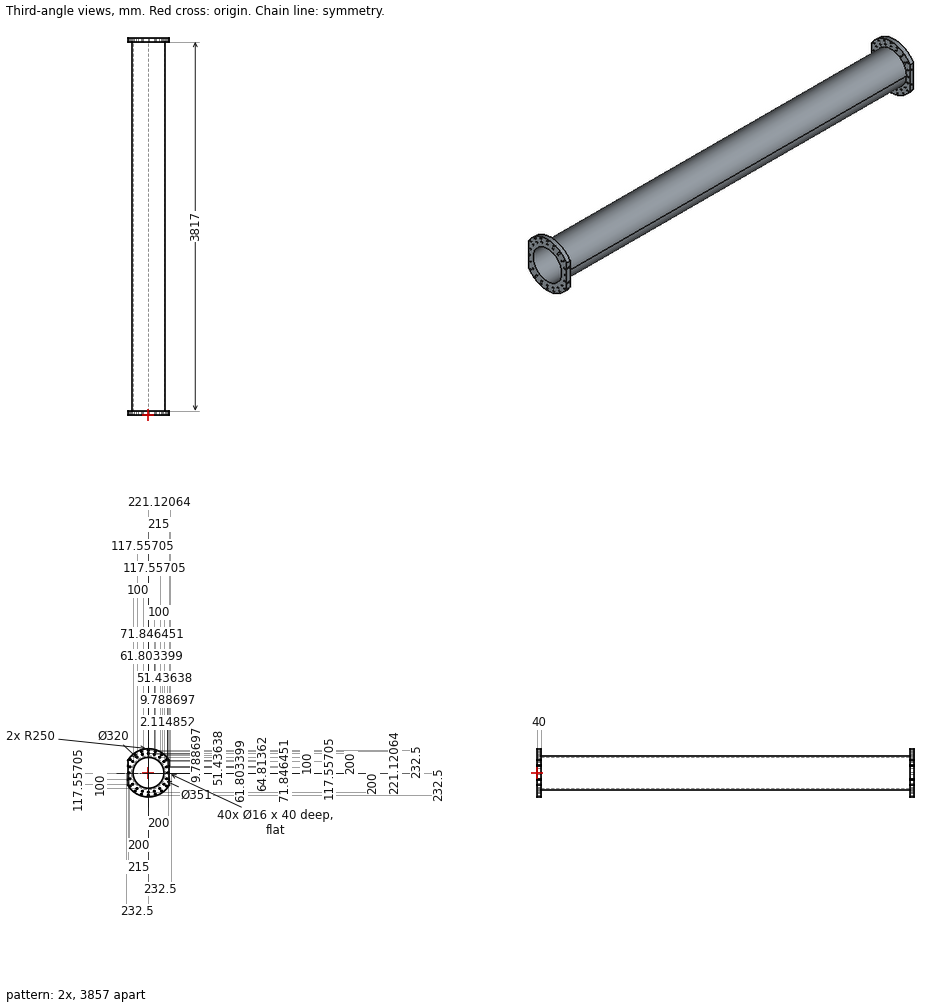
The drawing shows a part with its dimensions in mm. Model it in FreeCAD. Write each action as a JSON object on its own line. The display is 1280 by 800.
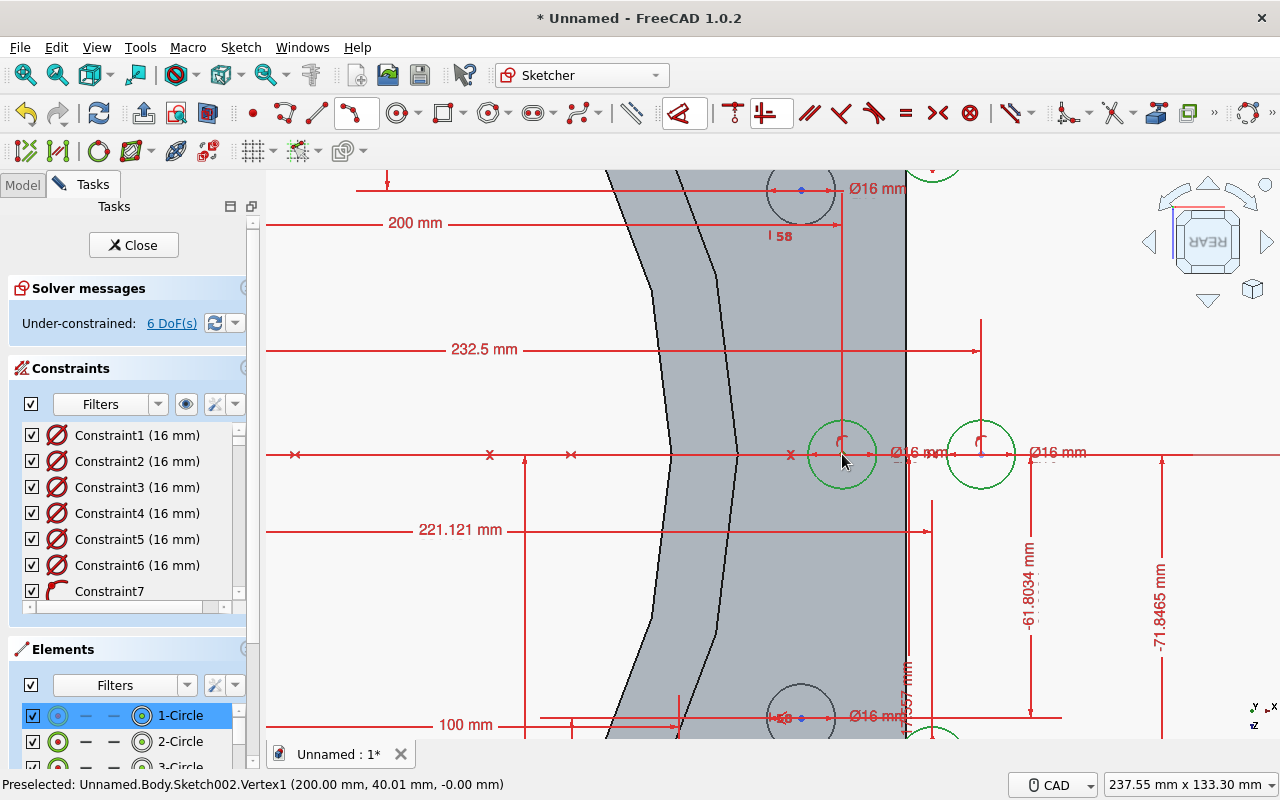
{"action": "scroll", "coordinate": [846, 455], "scroll_direction": "down", "scroll_amount": 9}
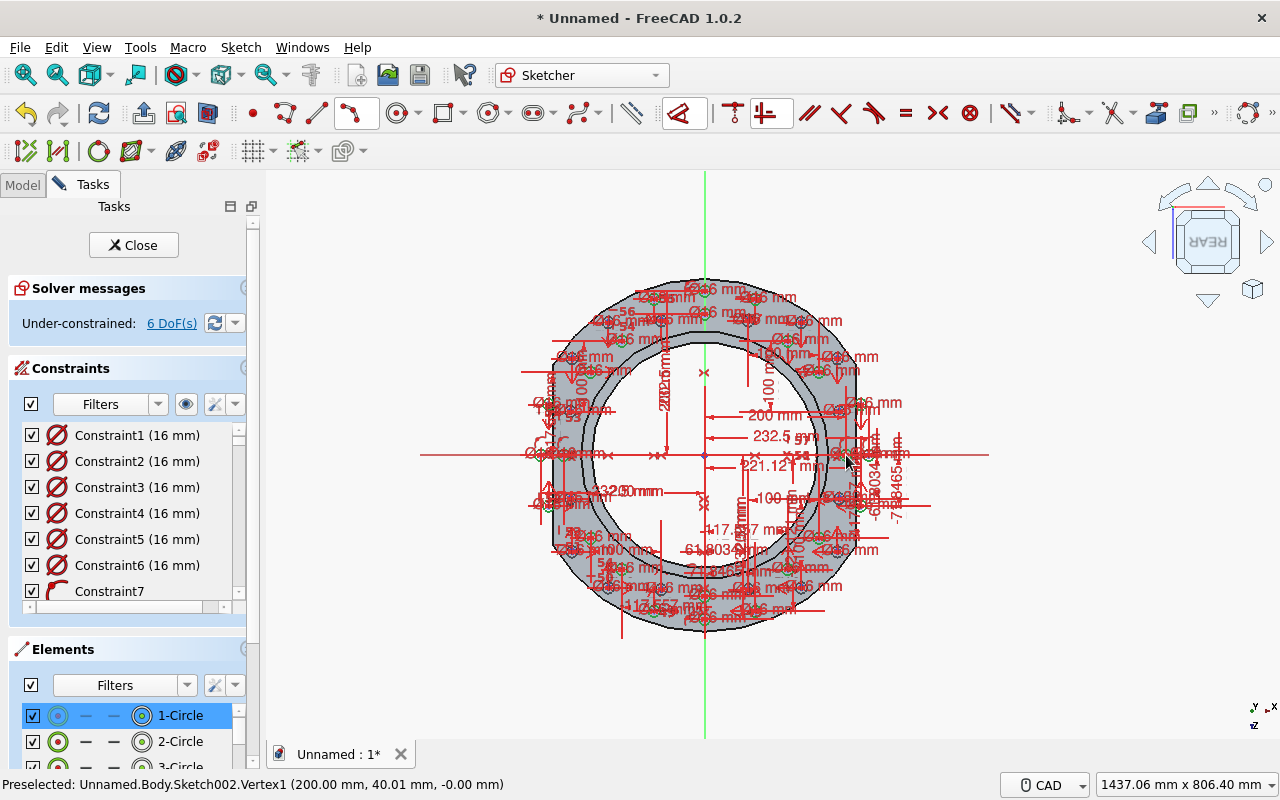
{"action": "scroll", "coordinate": [839, 499], "scroll_direction": "up", "scroll_amount": 9}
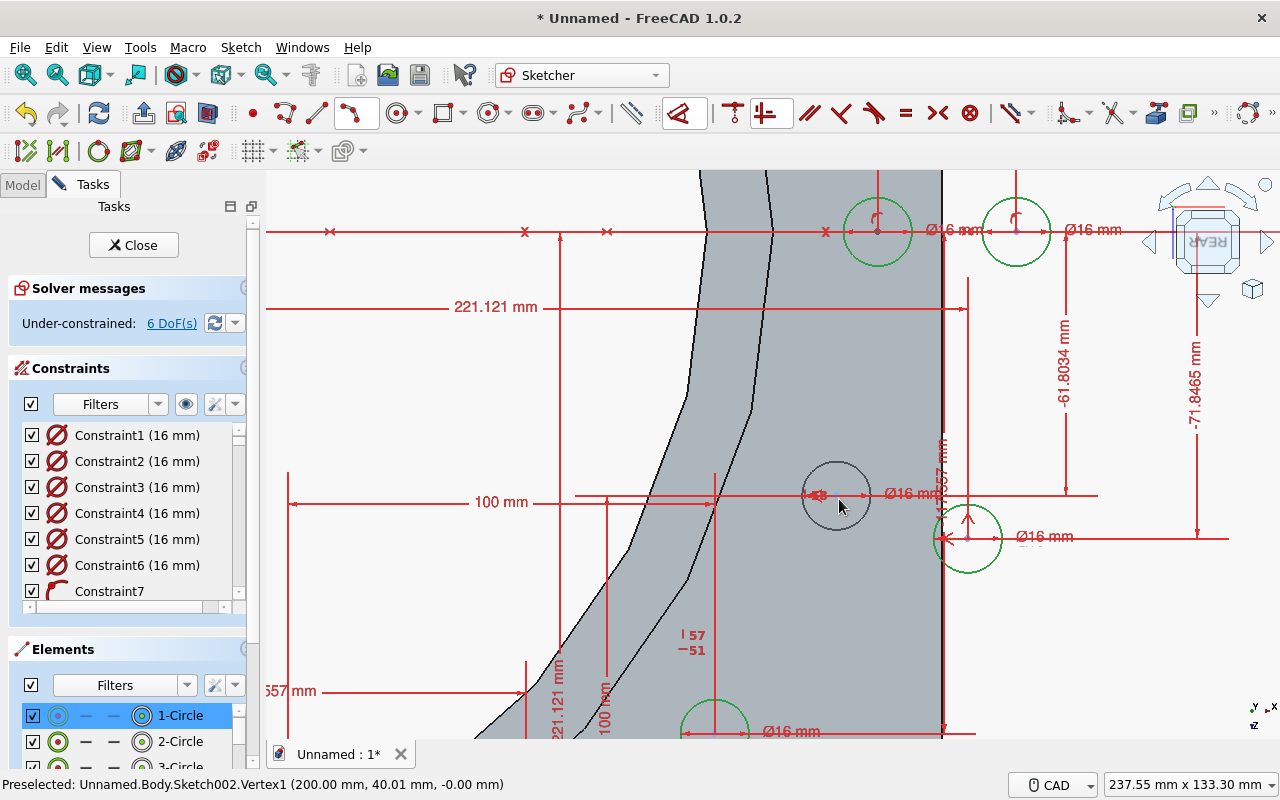
{"action": "left_click", "coordinate": [836, 496]}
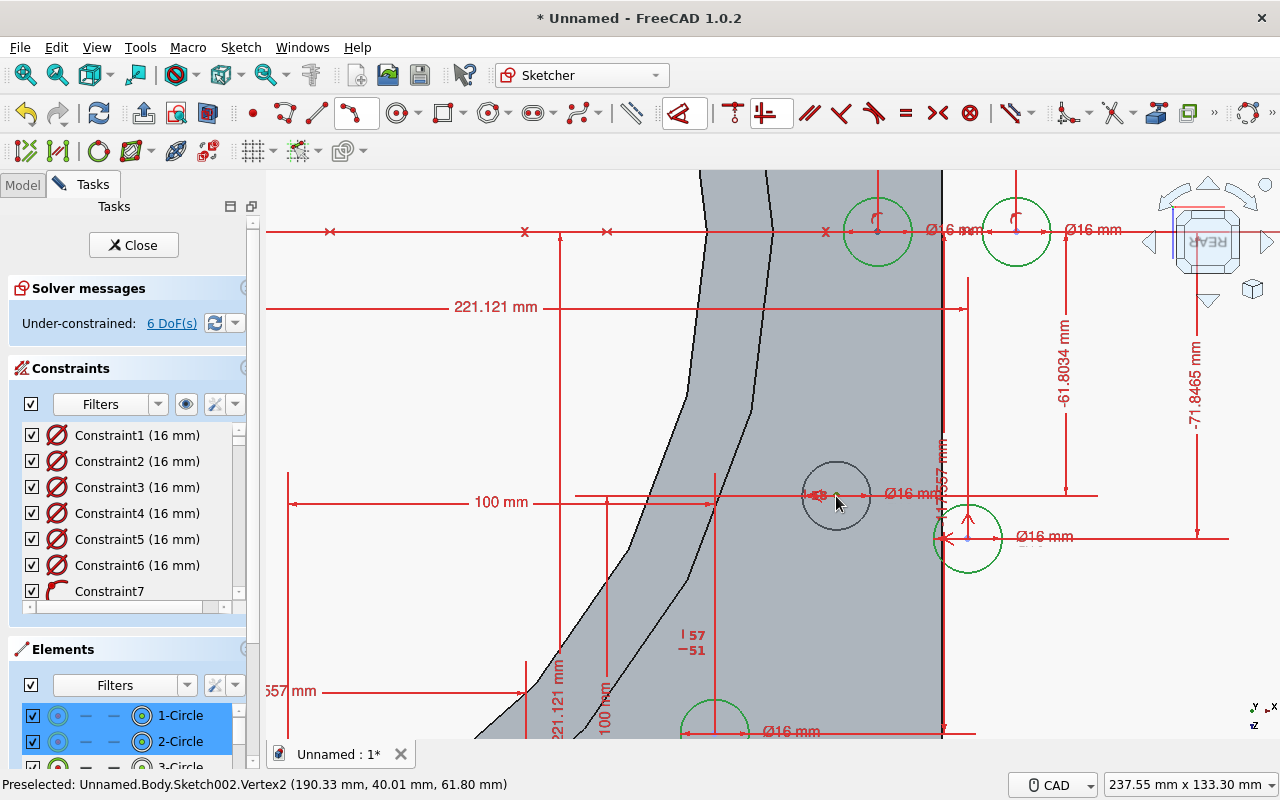
{"action": "left_click", "coordinate": [702, 114]}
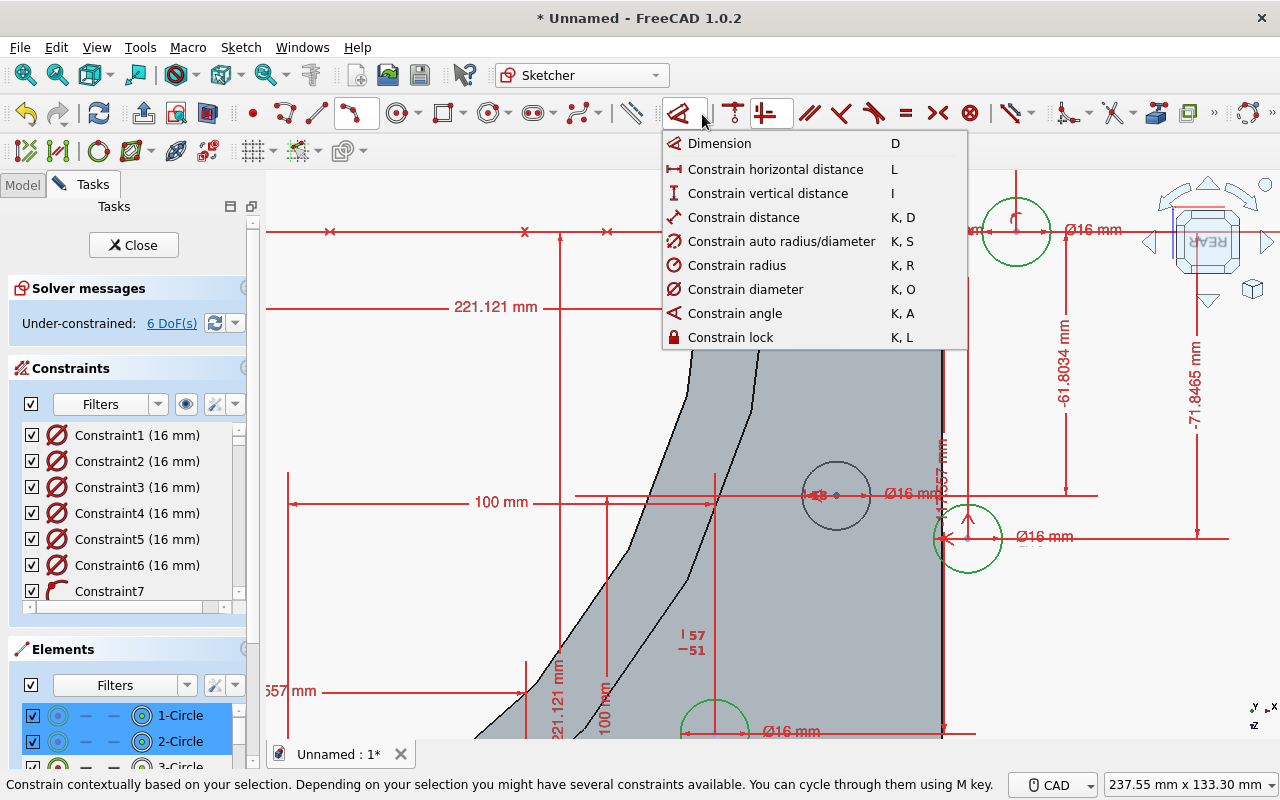
{"action": "left_click", "coordinate": [815, 169]}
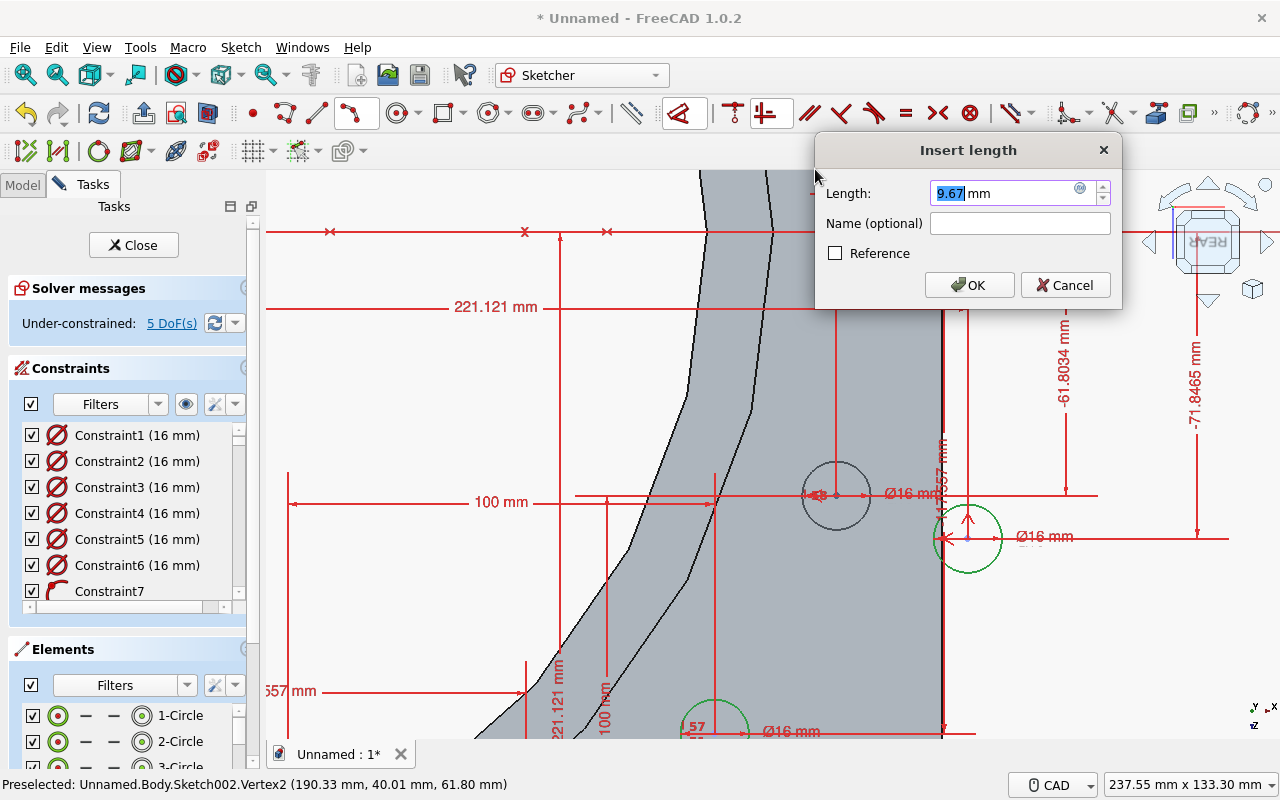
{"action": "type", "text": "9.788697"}
{"action": "key", "text": "Return"}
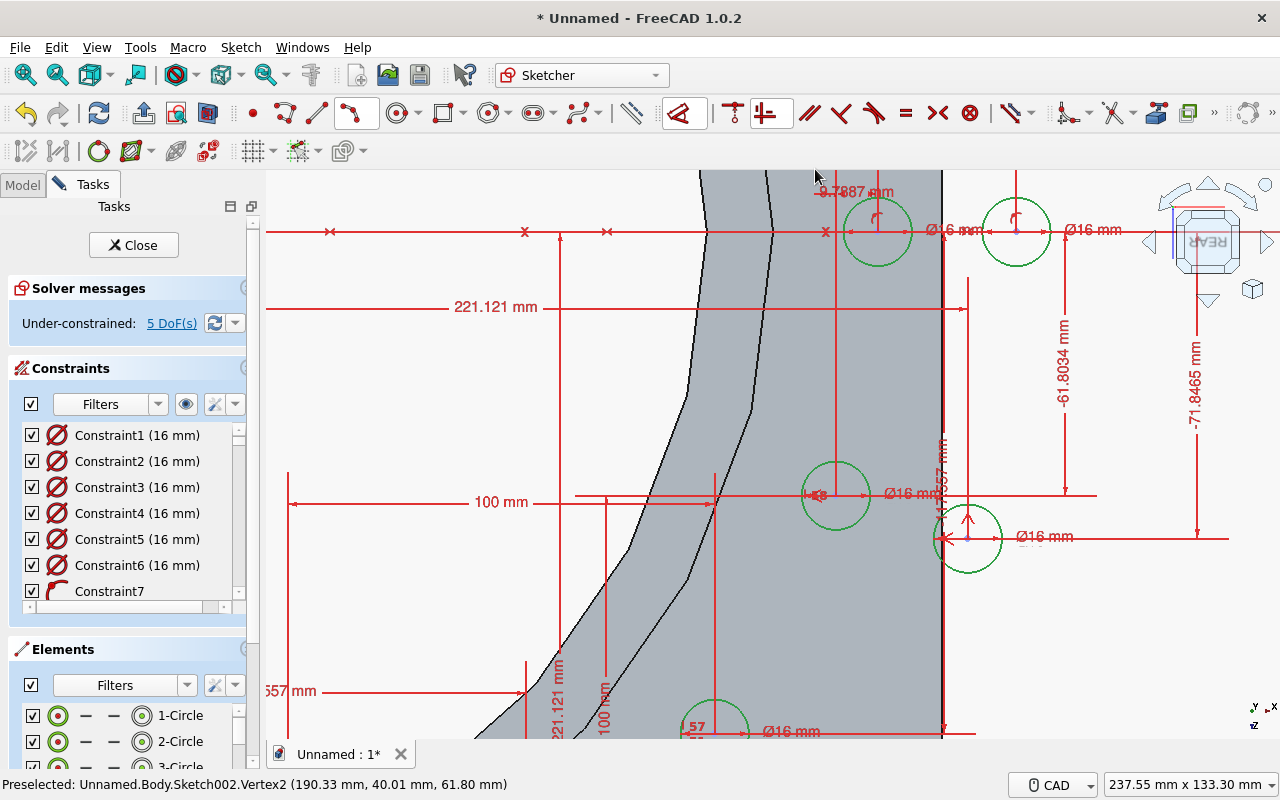
{"action": "scroll", "coordinate": [839, 499], "scroll_direction": "down", "scroll_amount": 9}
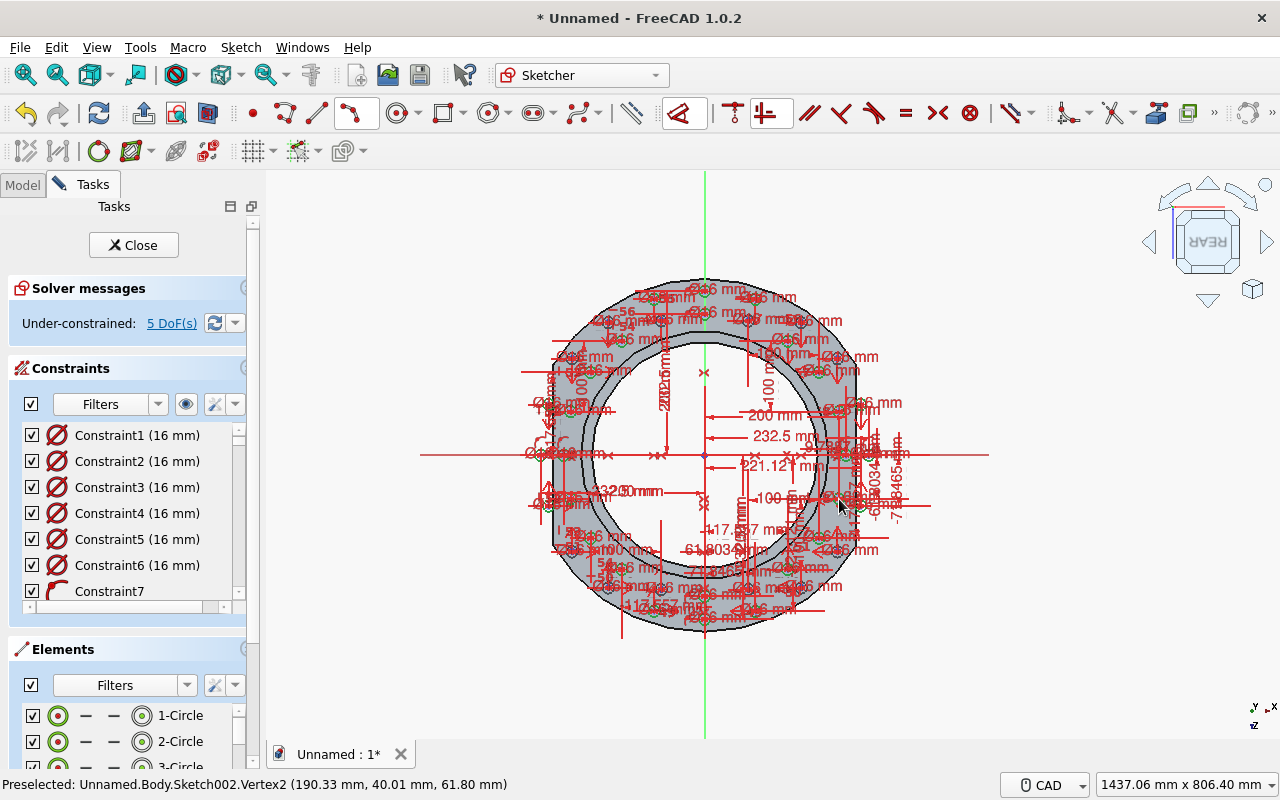
{"action": "scroll", "coordinate": [748, 590], "scroll_direction": "up", "scroll_amount": 9}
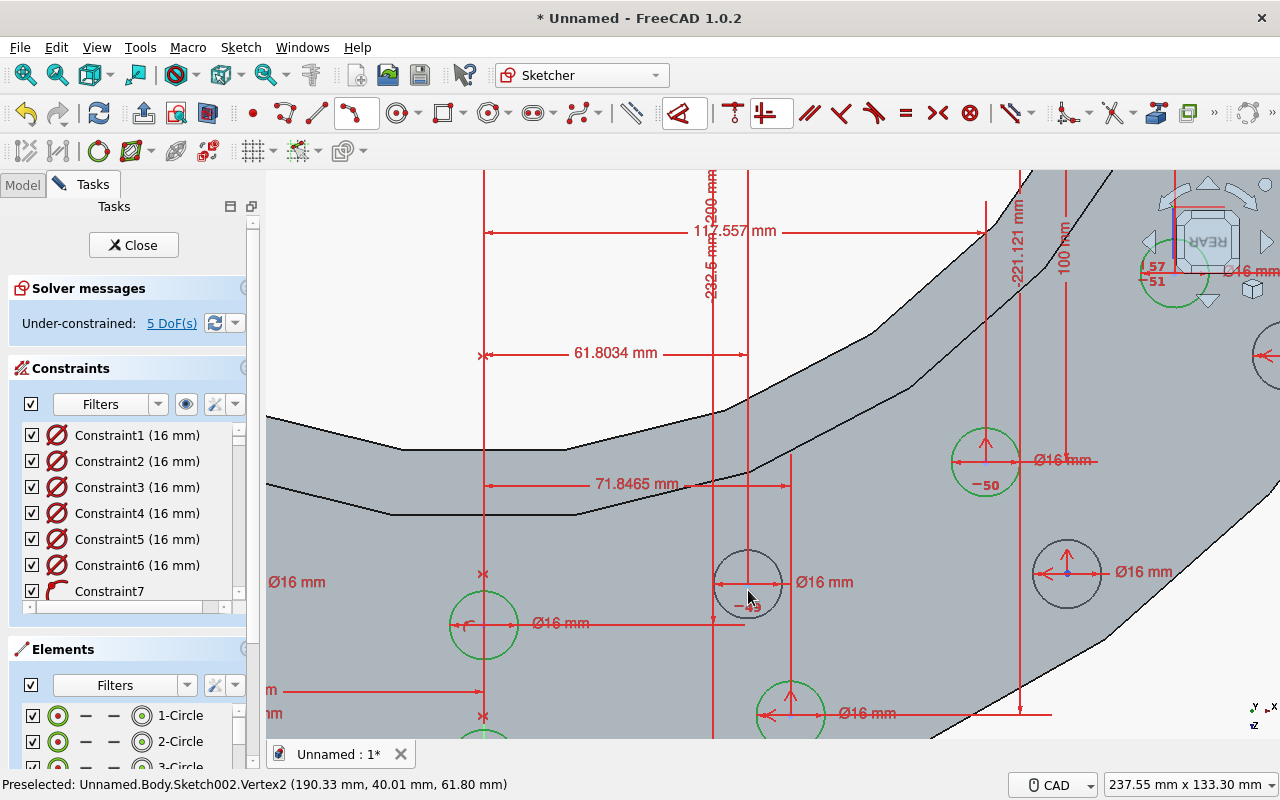
{"action": "left_click", "coordinate": [748, 584]}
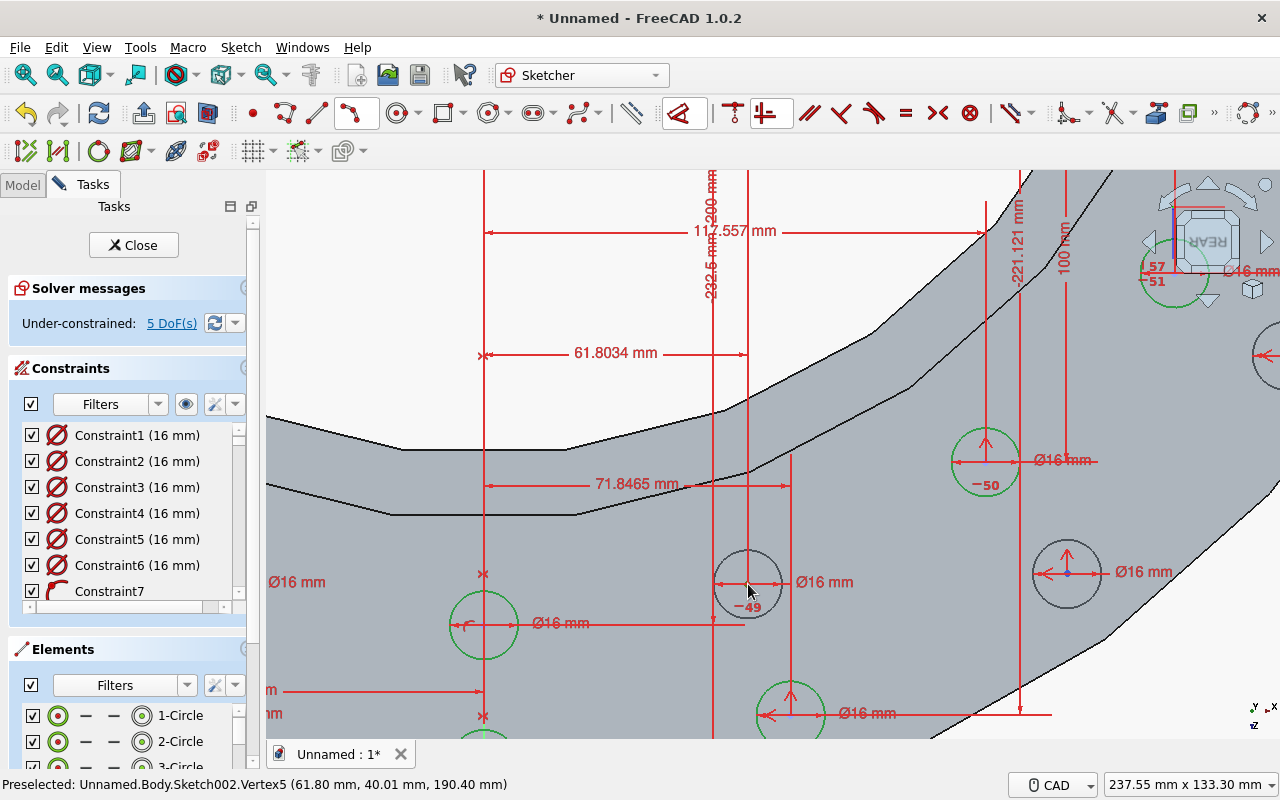
{"action": "left_click", "coordinate": [484, 625]}